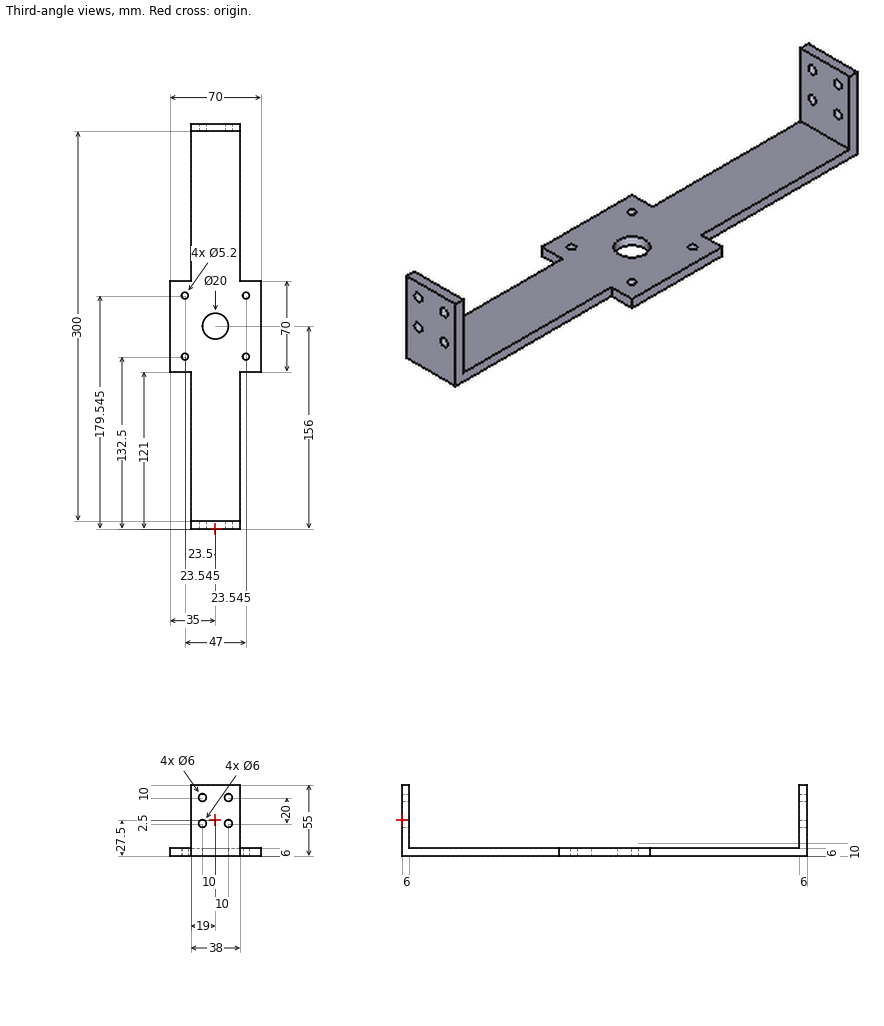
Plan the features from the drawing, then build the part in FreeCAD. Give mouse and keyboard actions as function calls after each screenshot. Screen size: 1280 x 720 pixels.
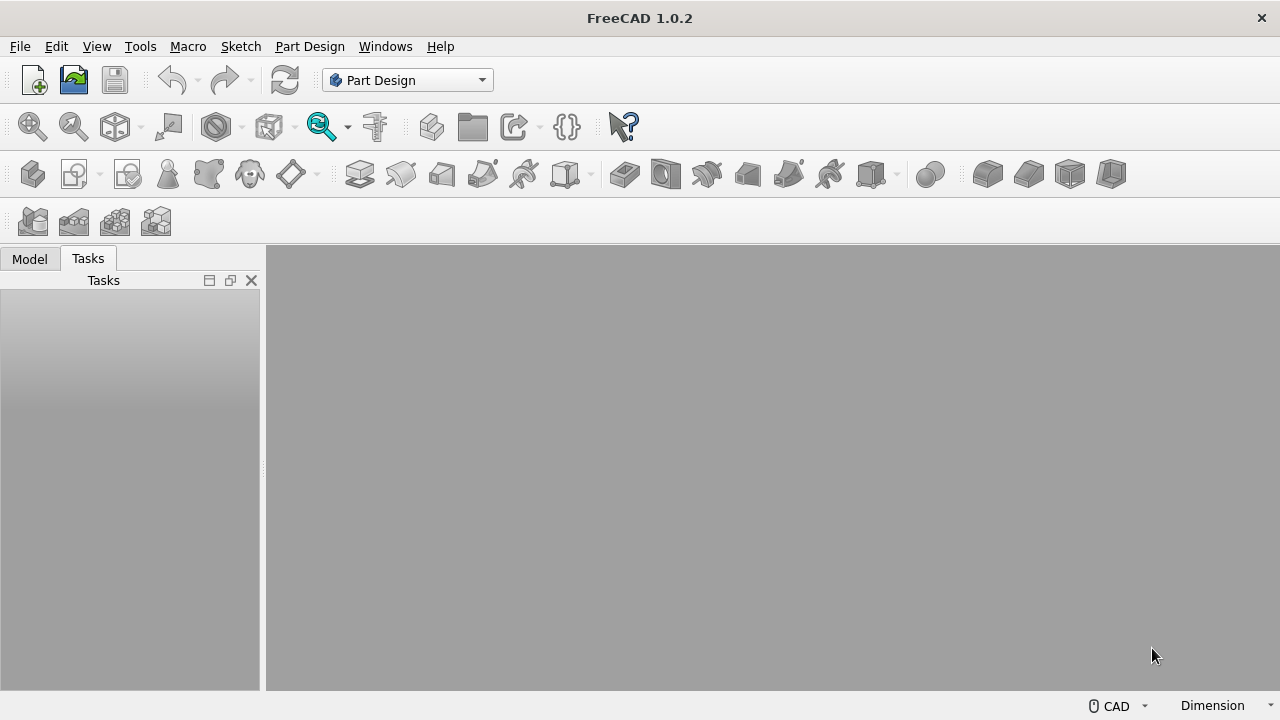
key(ctrl+n)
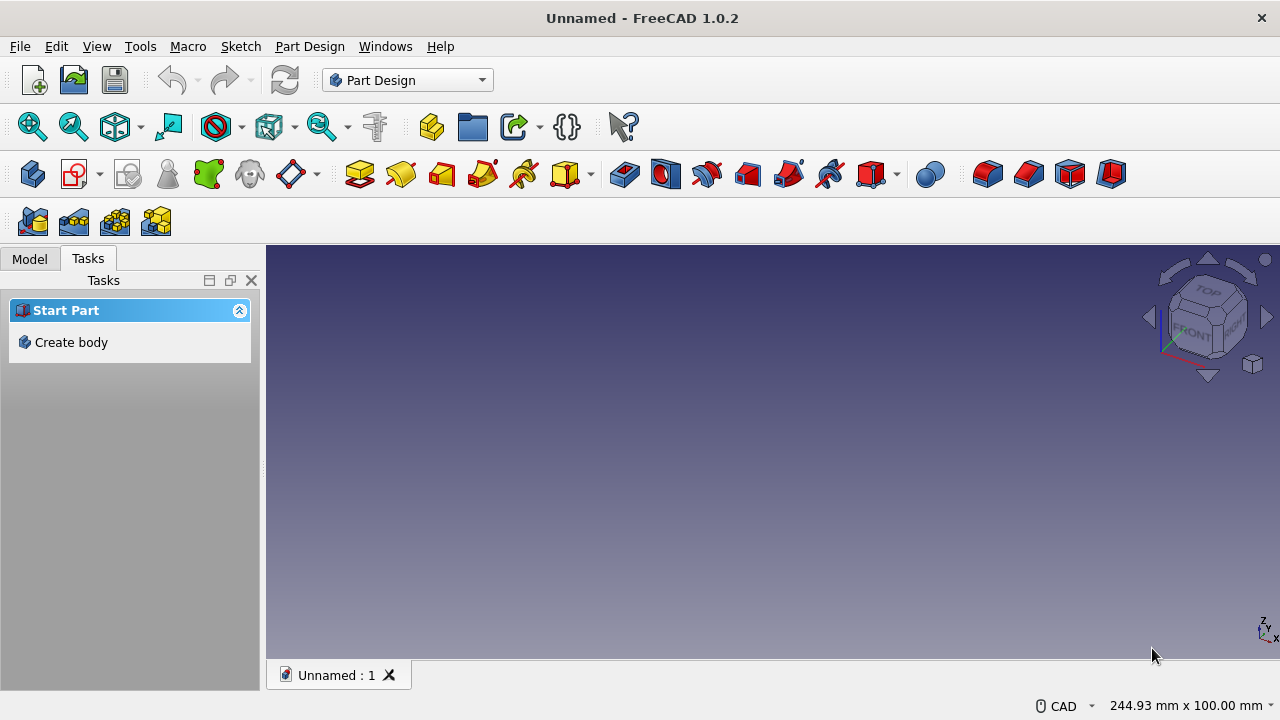
click(74, 174)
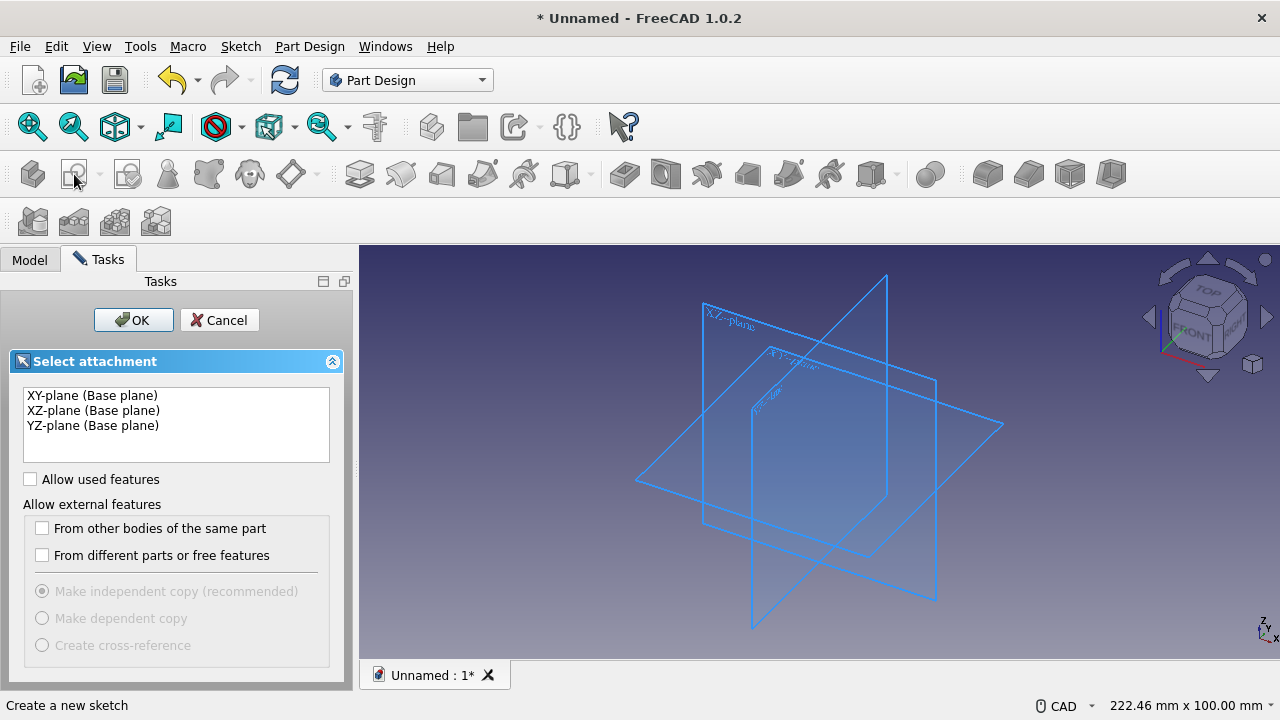
click(84, 410)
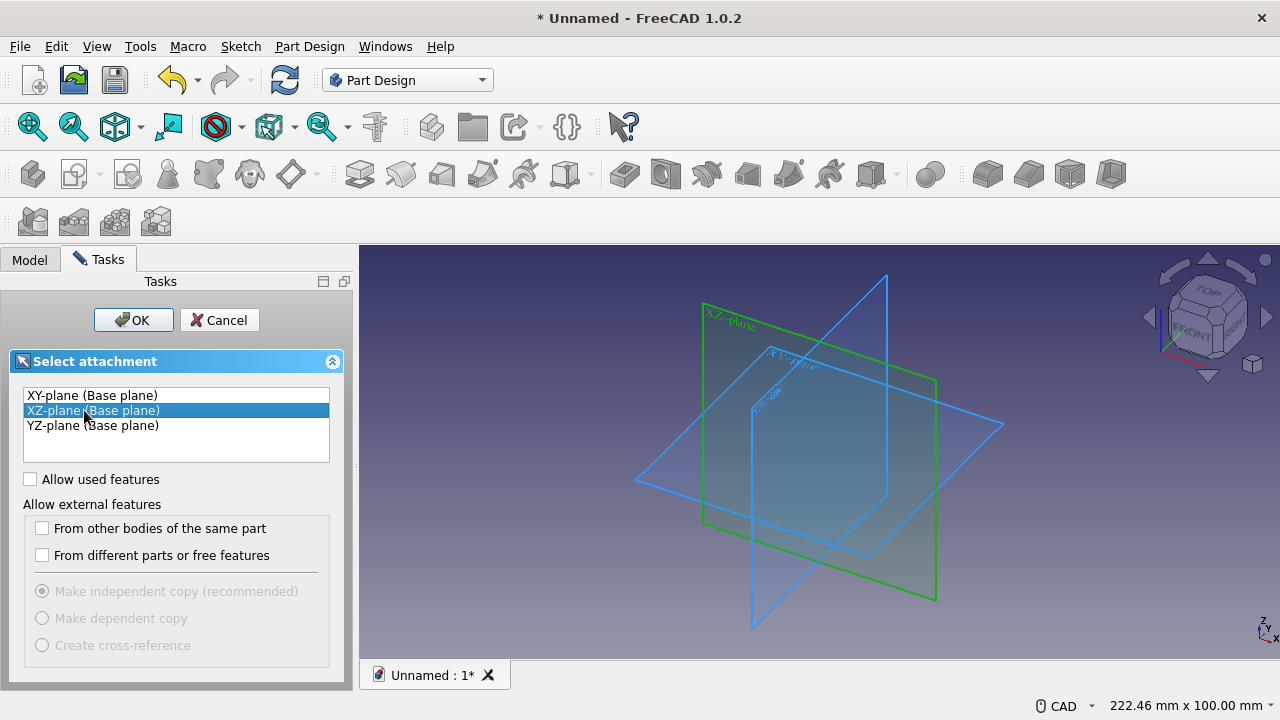
click(134, 320)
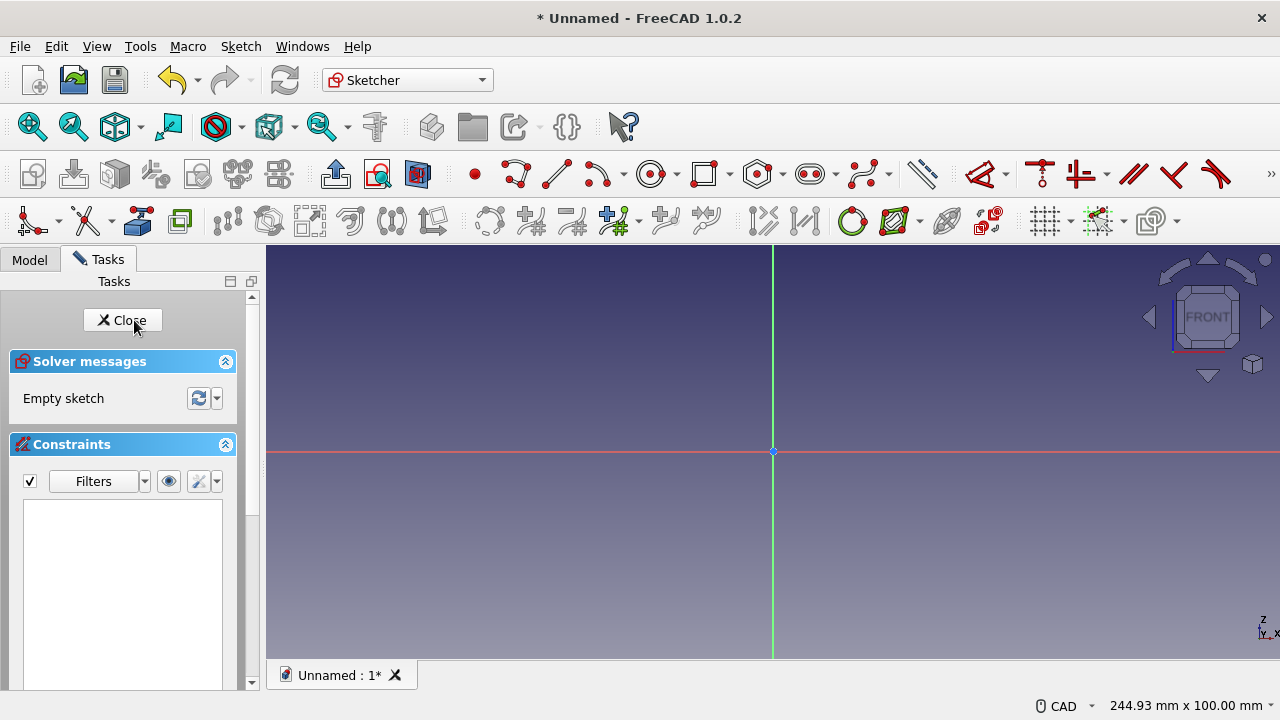
key(g)
key(v)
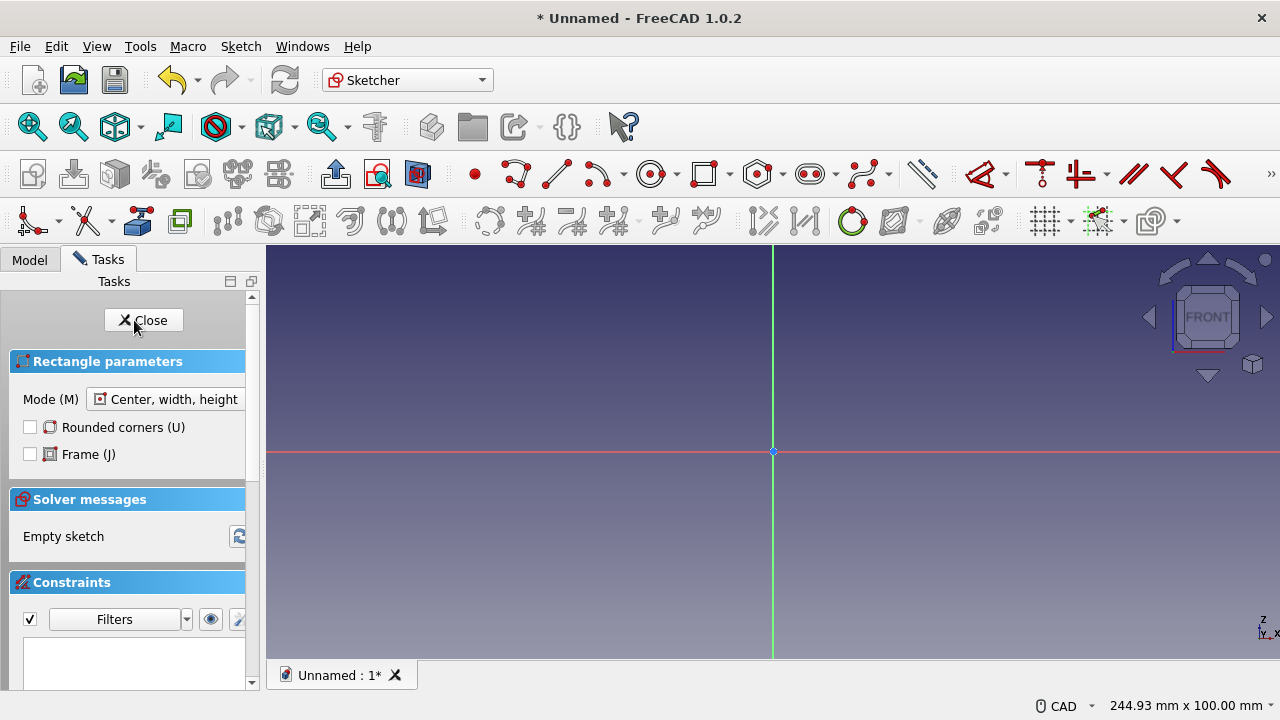
click(773, 452)
move(852, 338)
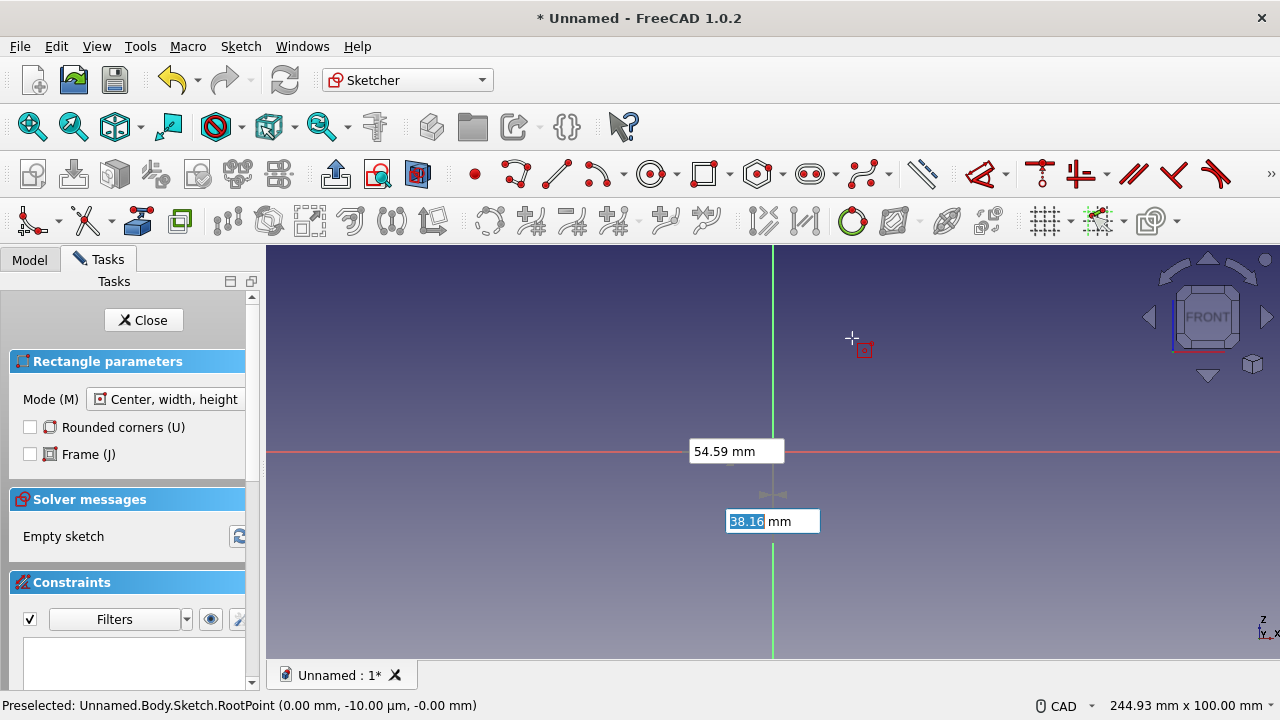
text(38)
key(Tab)
text(55)
key(Return)
key(Escape)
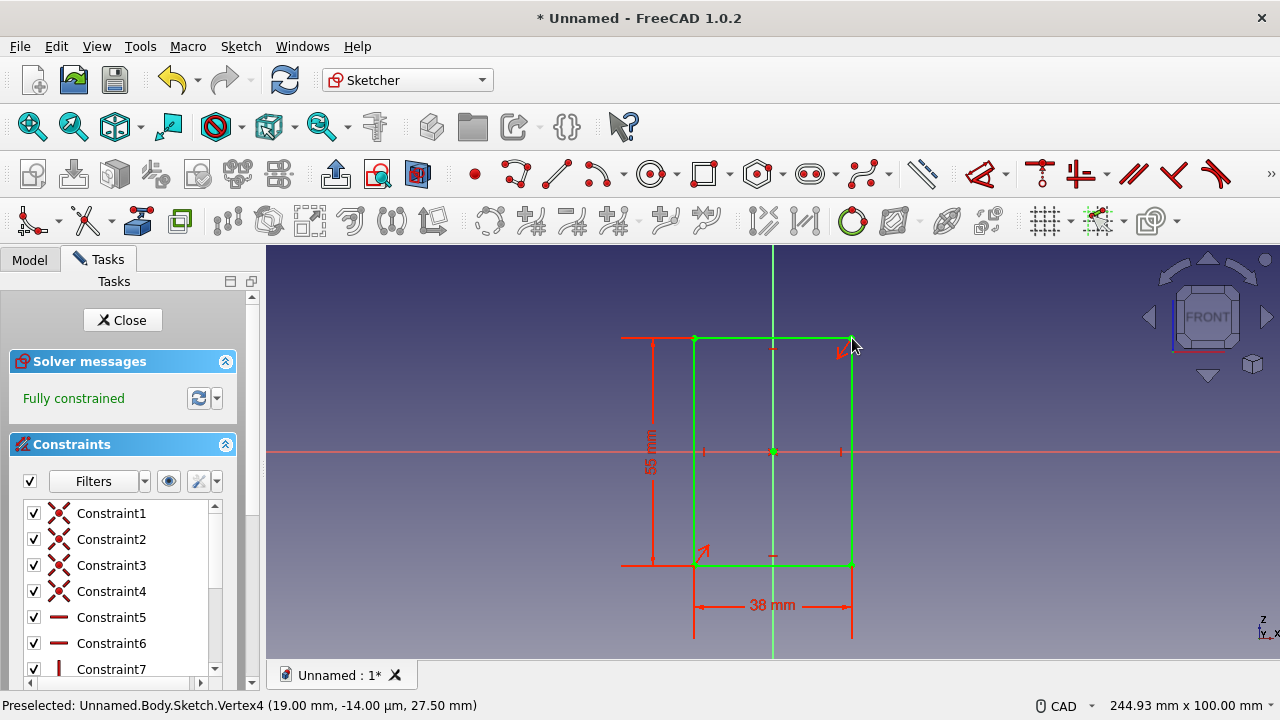
click(123, 320)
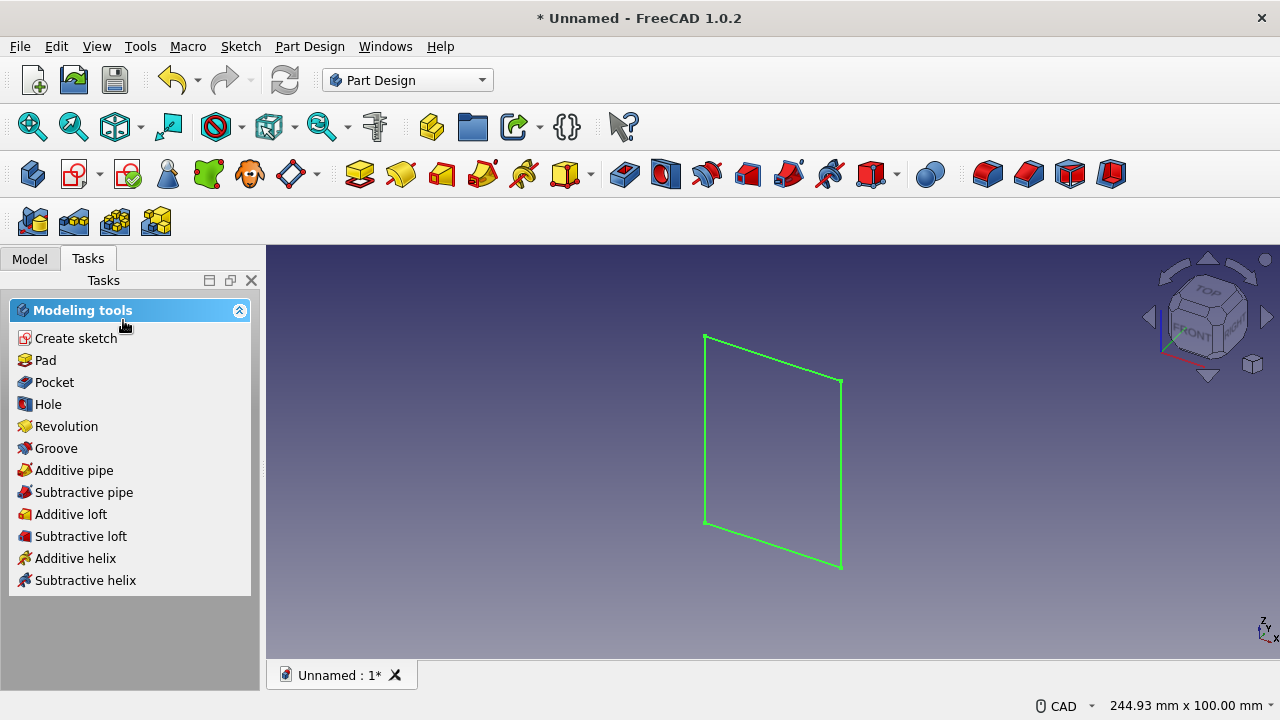
click(360, 174)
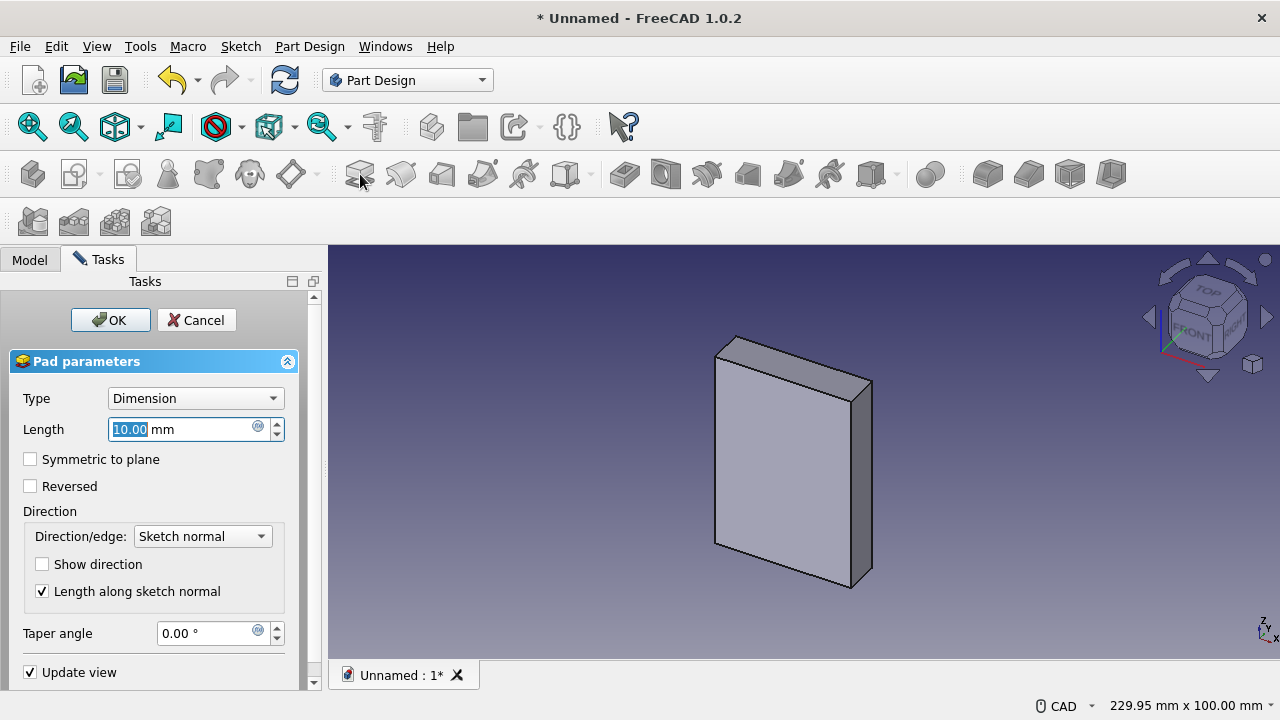
text(6)
key(Tab)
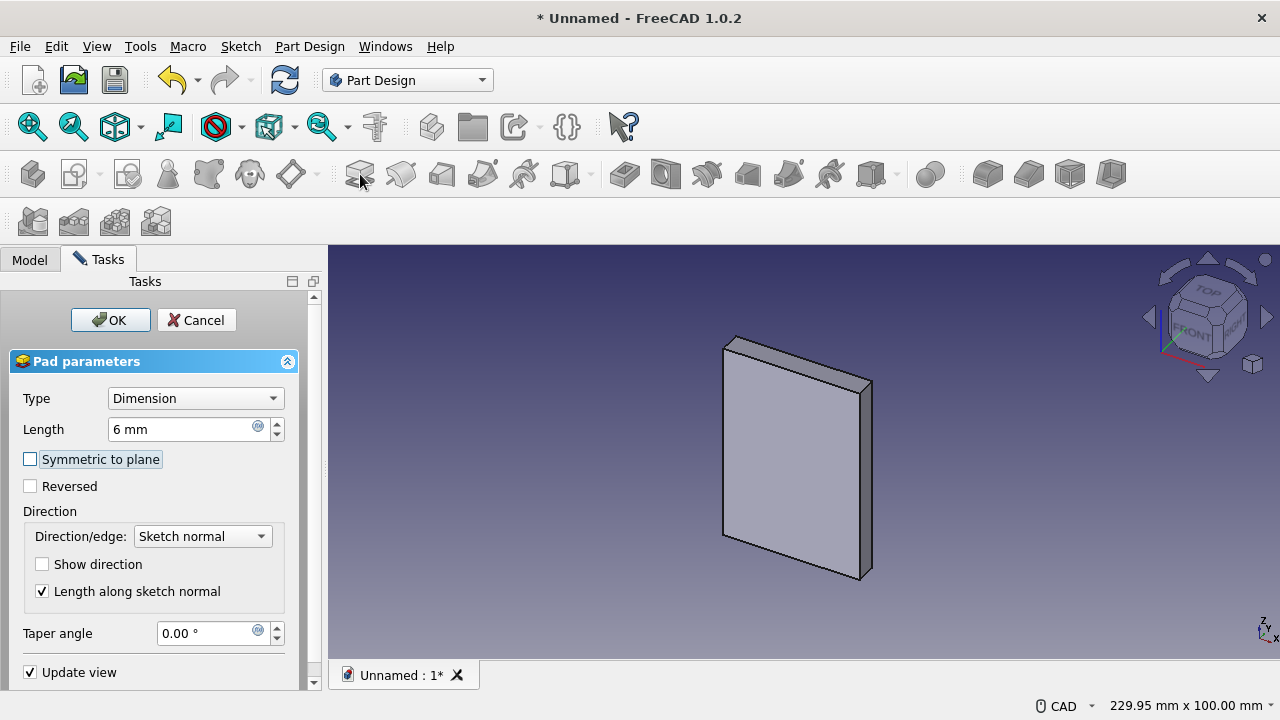
click(31, 486)